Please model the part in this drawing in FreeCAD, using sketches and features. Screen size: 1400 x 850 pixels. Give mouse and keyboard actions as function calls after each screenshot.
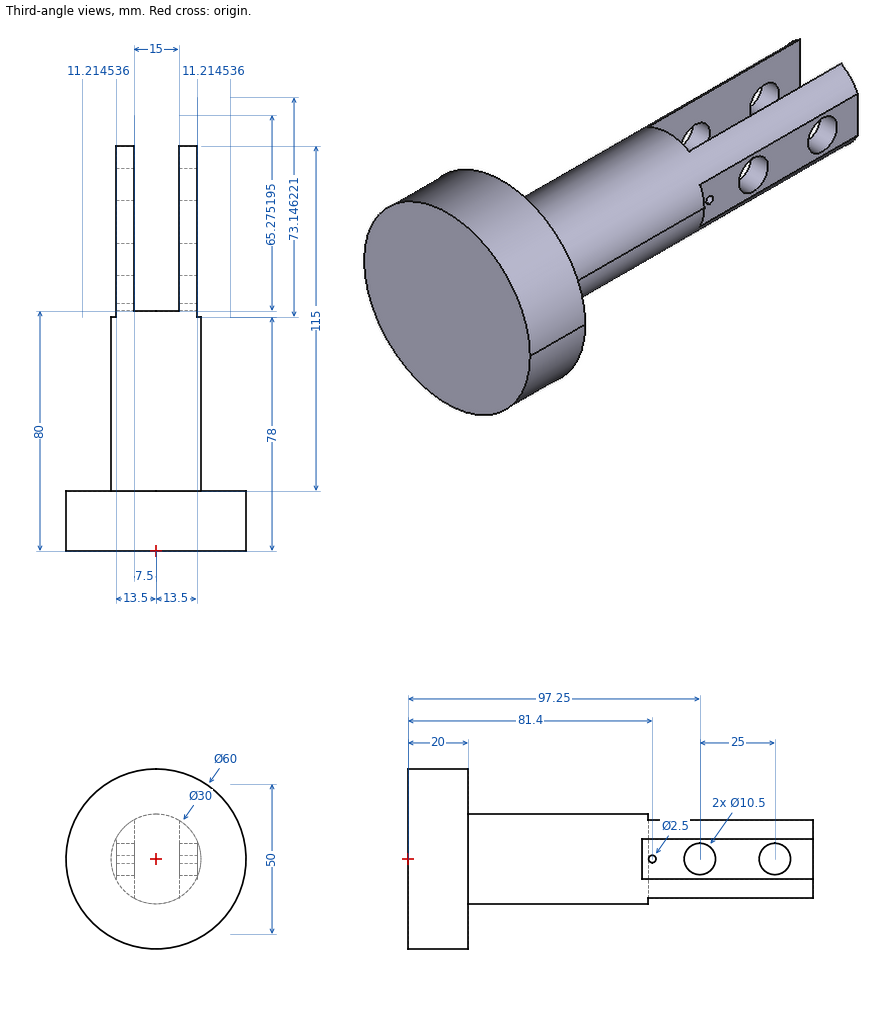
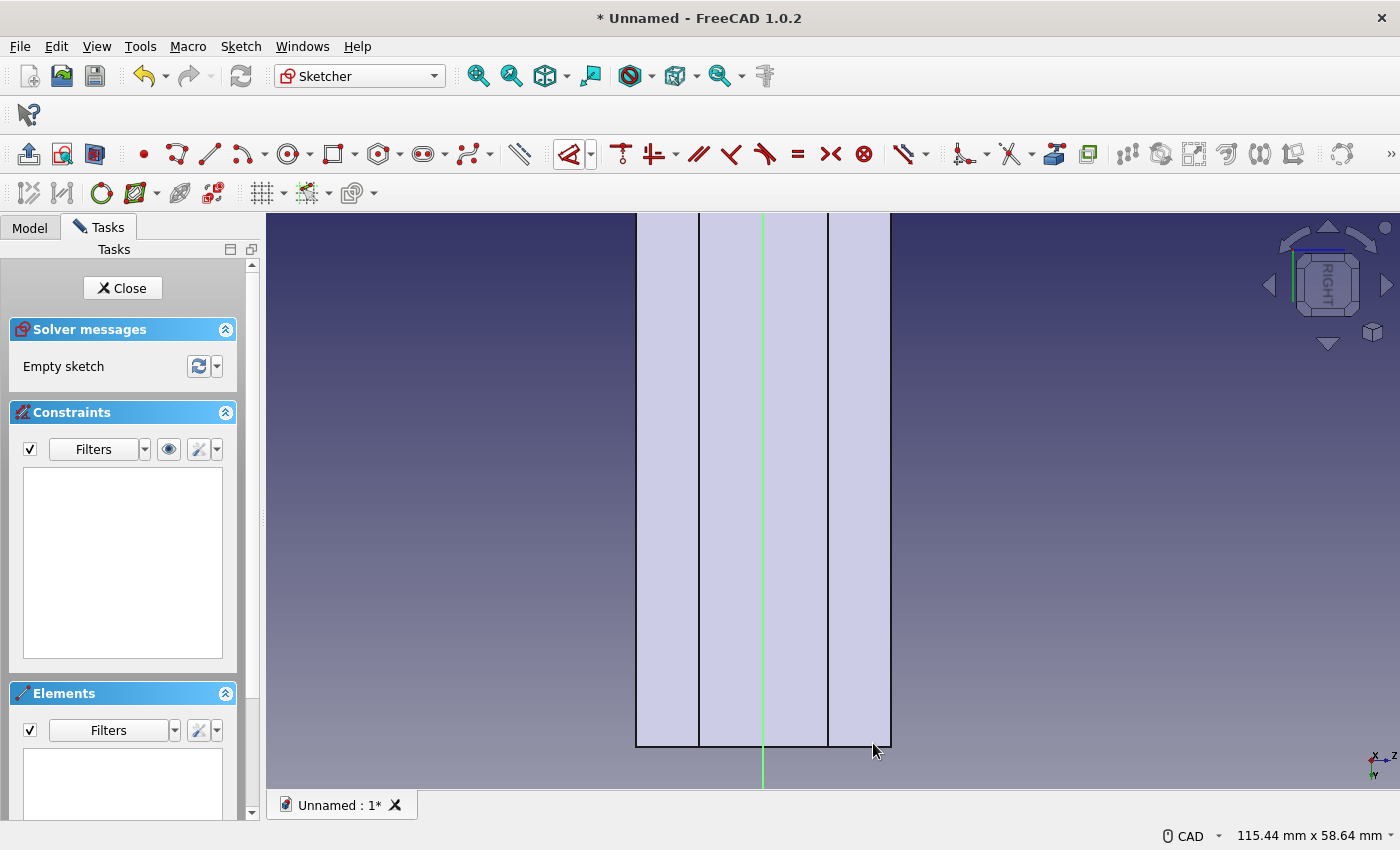
key(g)
key(c)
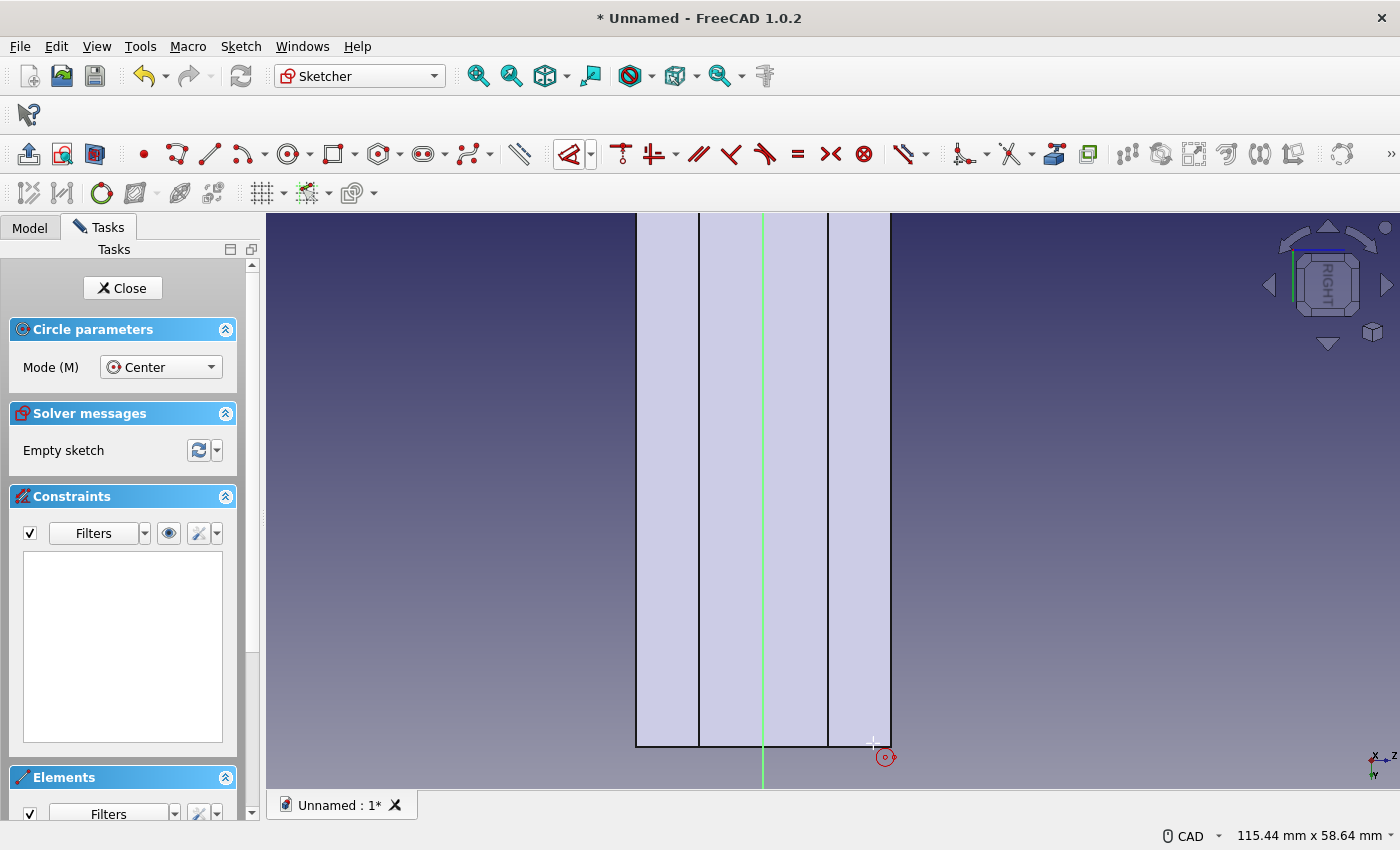
click(763, 376)
move(800, 339)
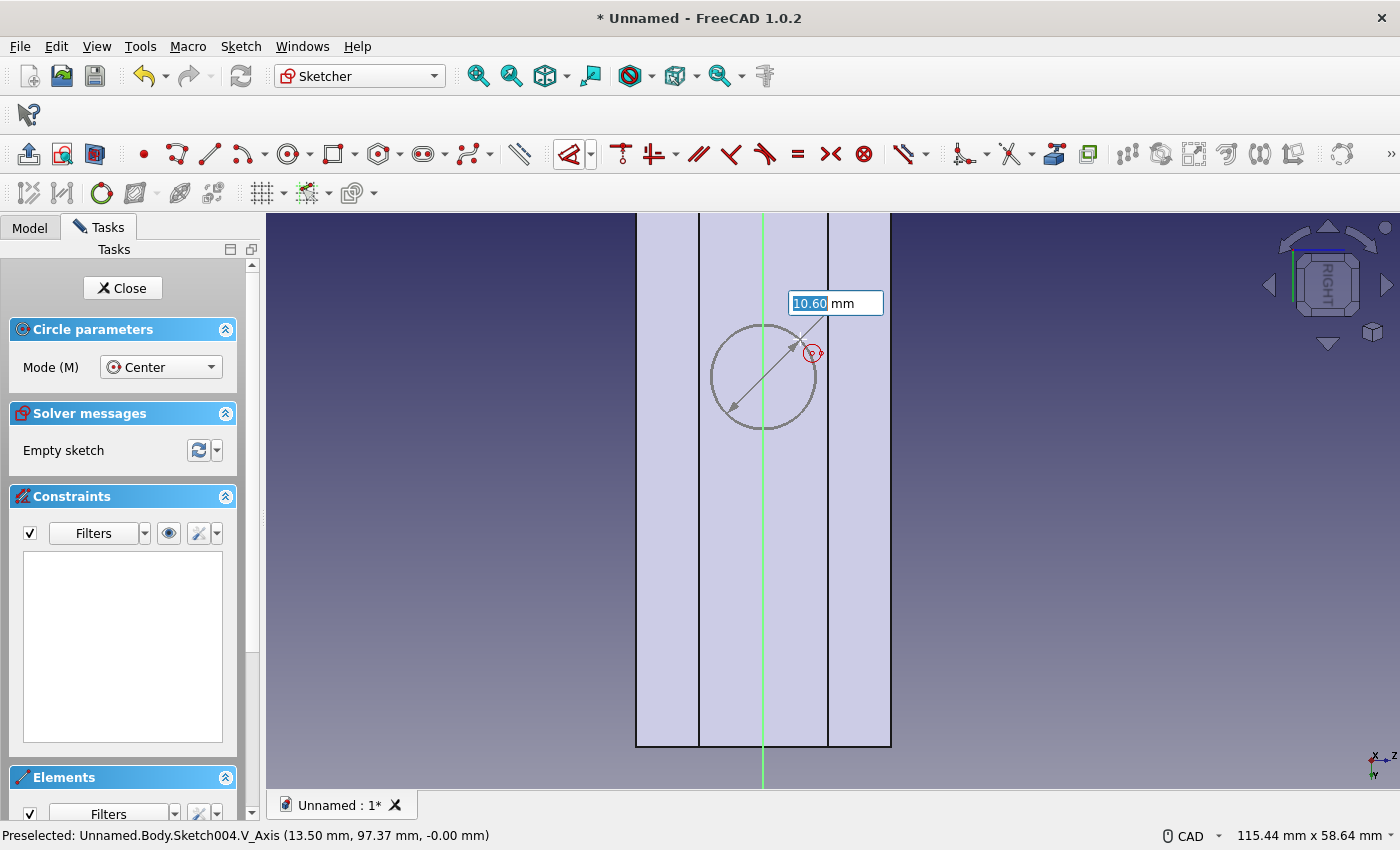
text(10.5)
key(Return)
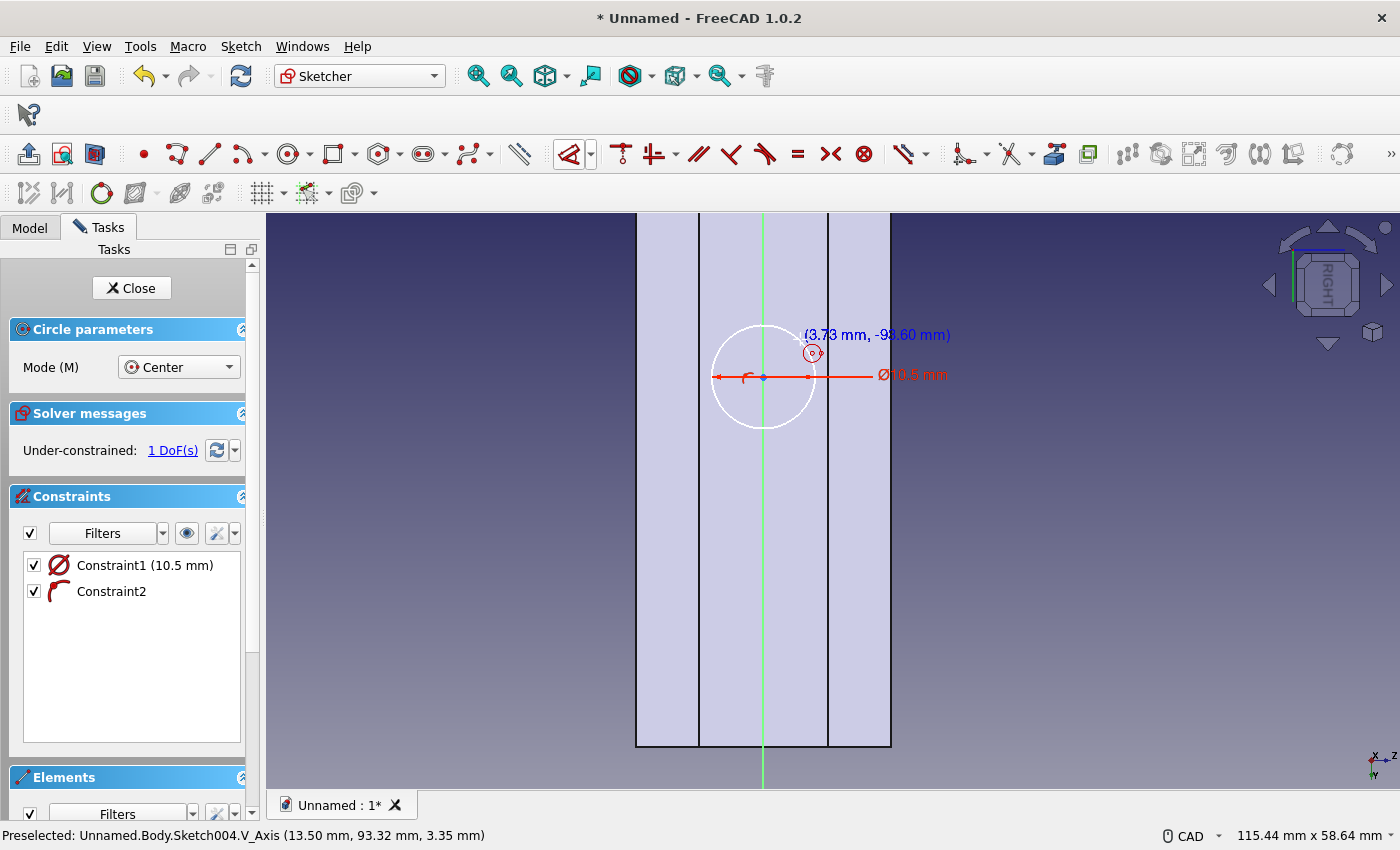
click(763, 621)
move(800, 585)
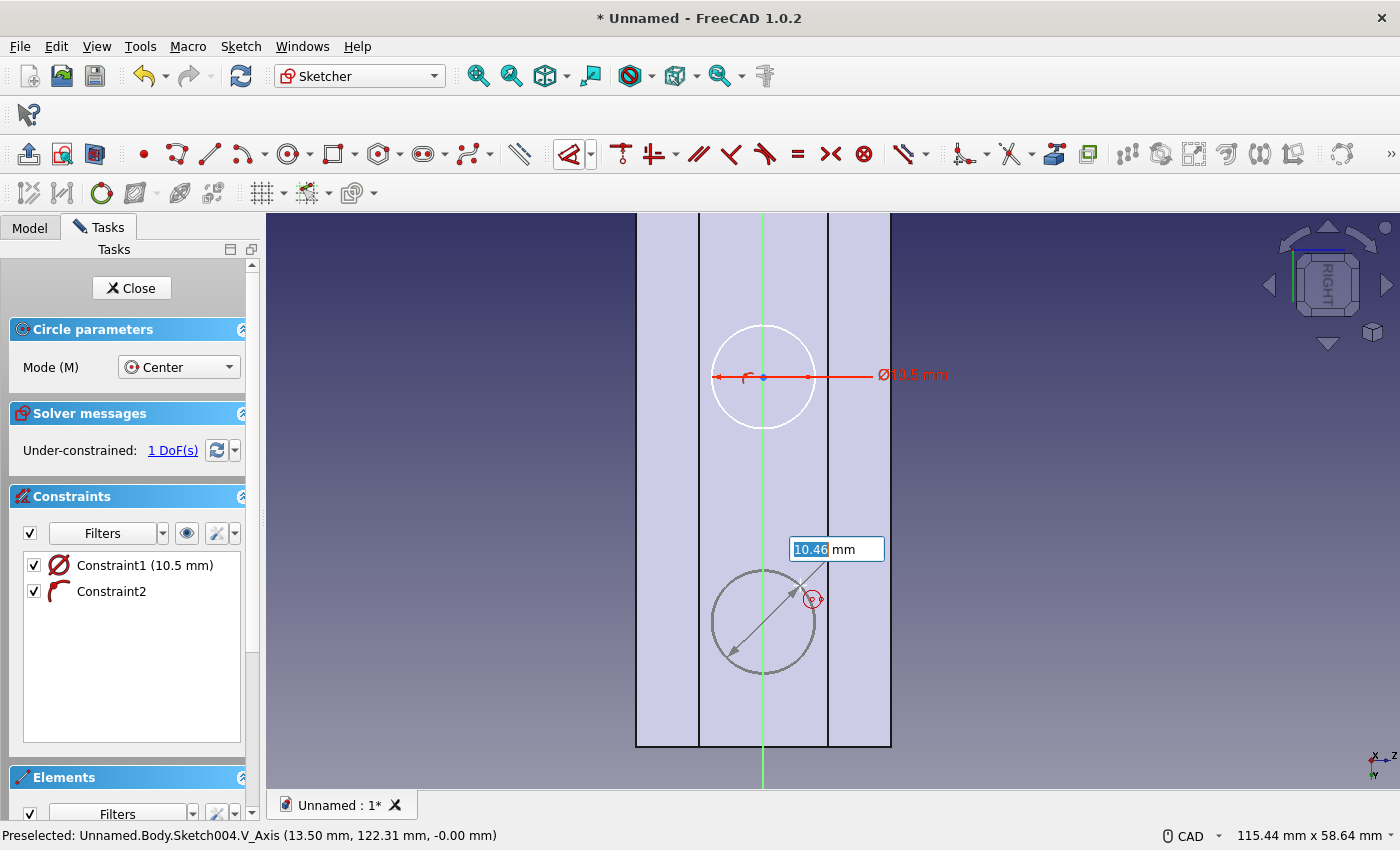
text(10.5)
key(Return)
key(Escape)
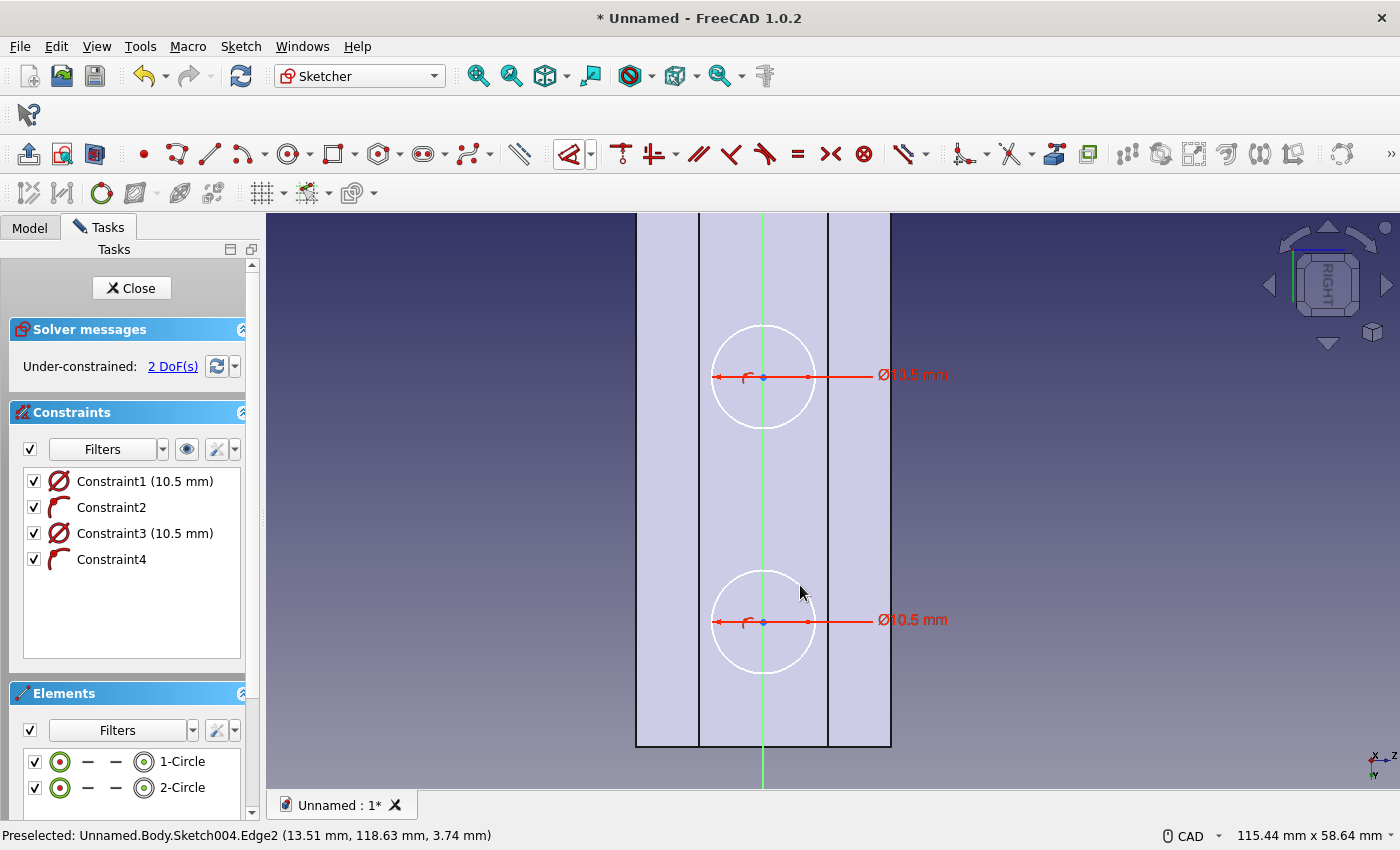
click(763, 377)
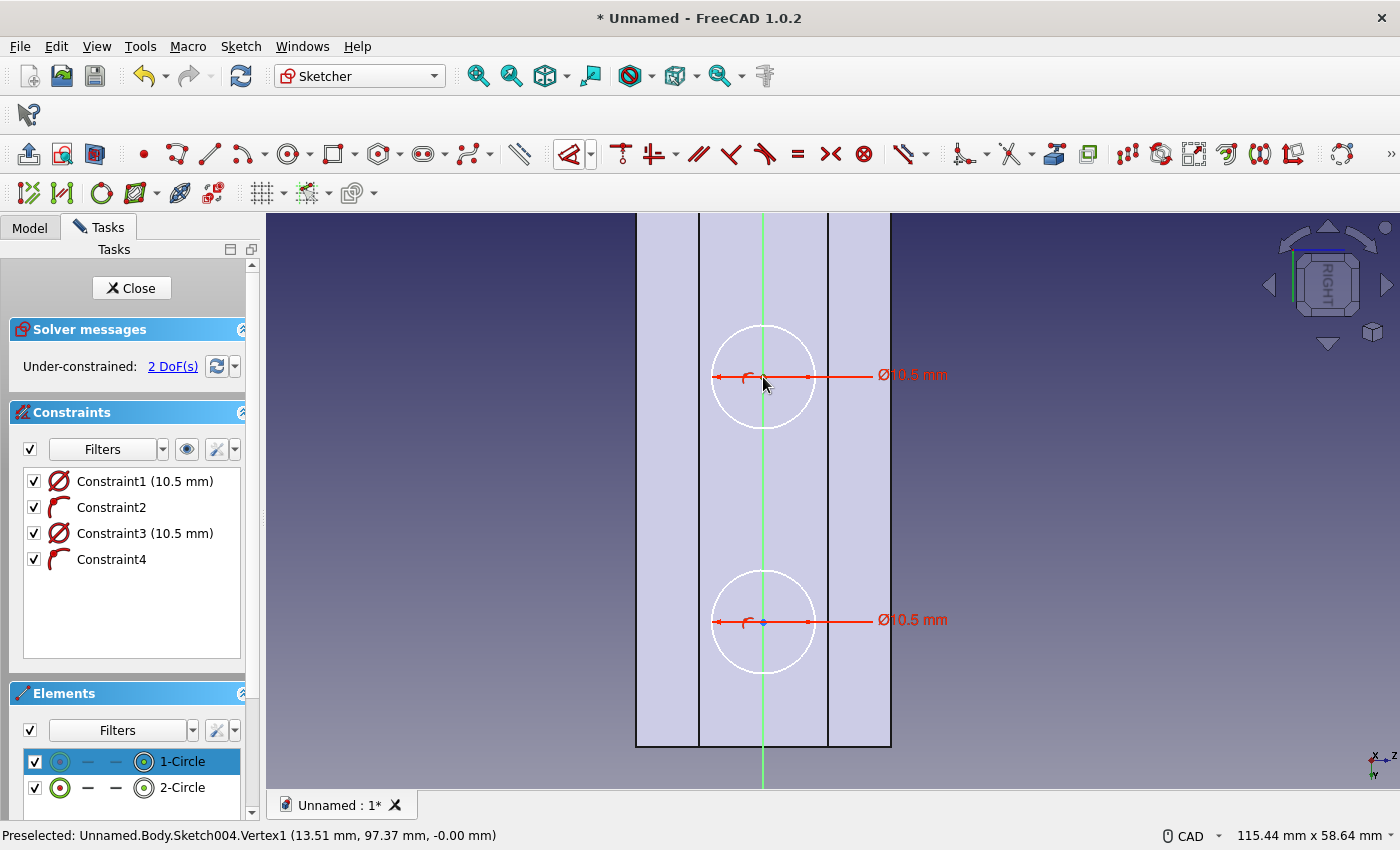
click(763, 622)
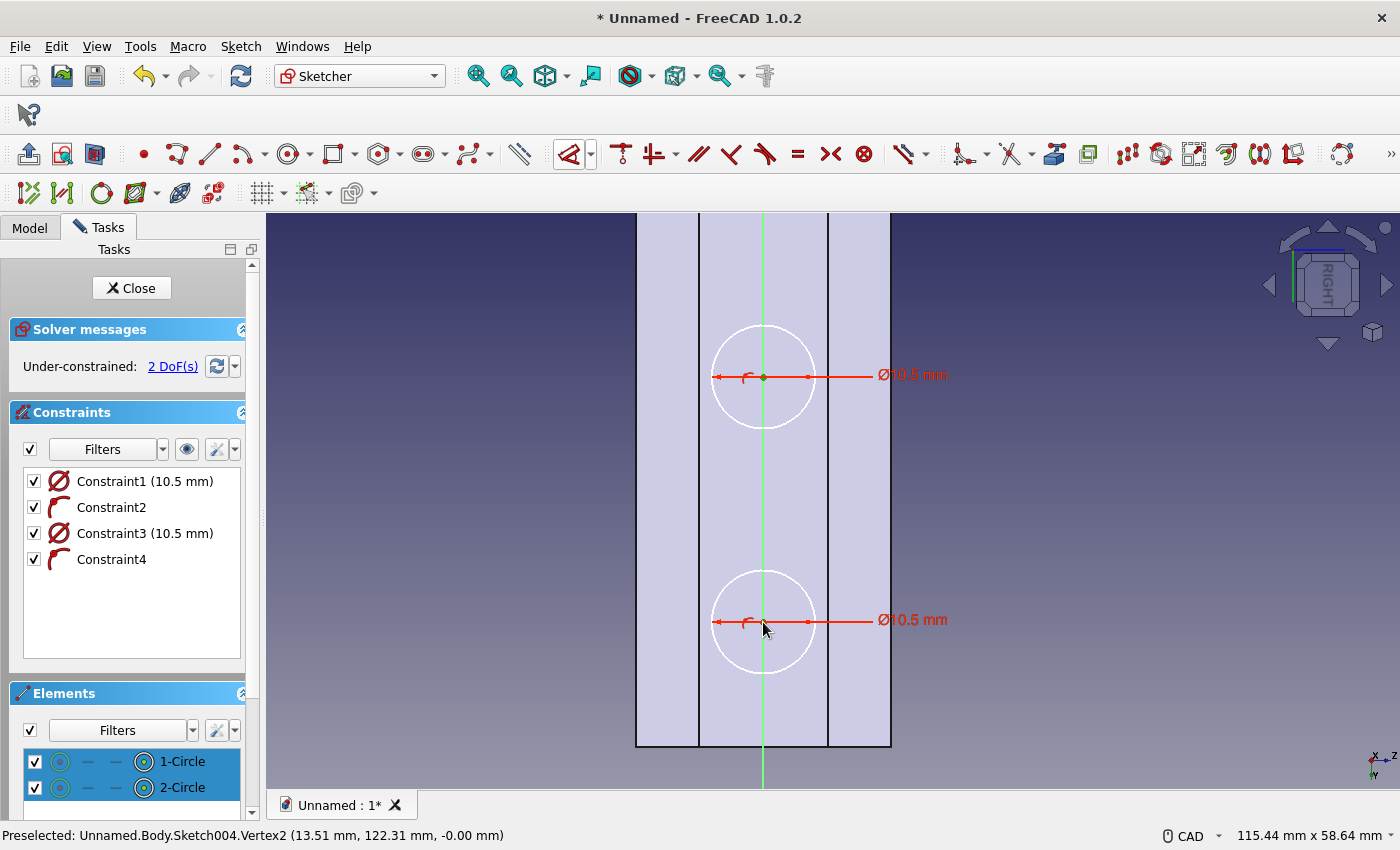
key(i)